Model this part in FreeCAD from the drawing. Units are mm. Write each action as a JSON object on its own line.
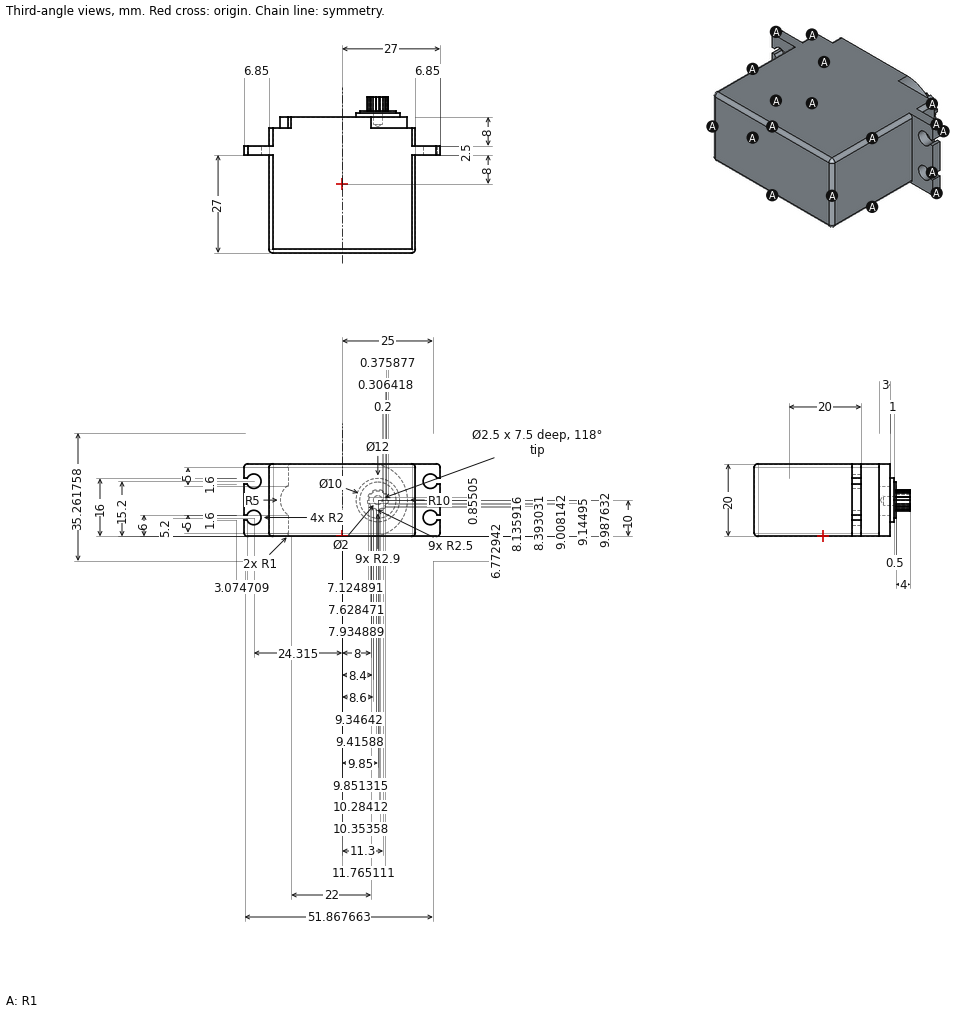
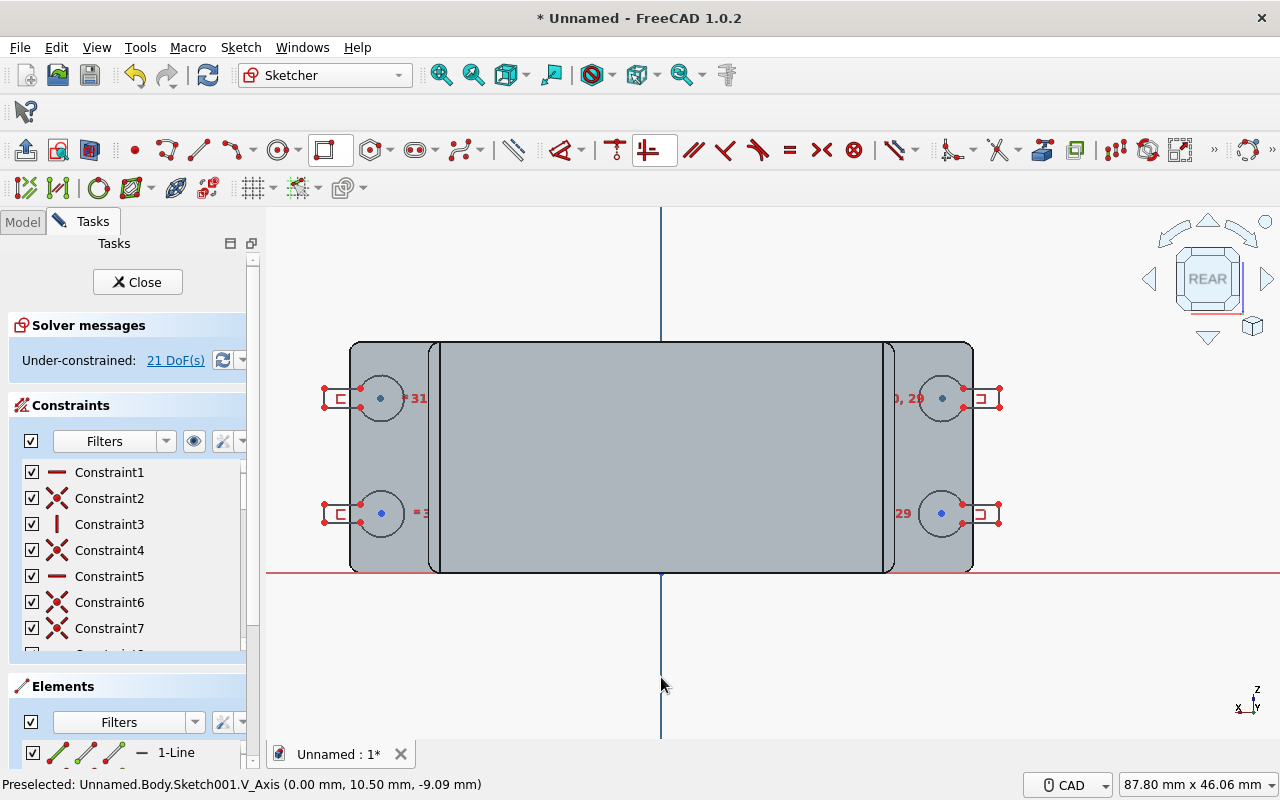
{"action": "left_click", "coordinate": [822, 150]}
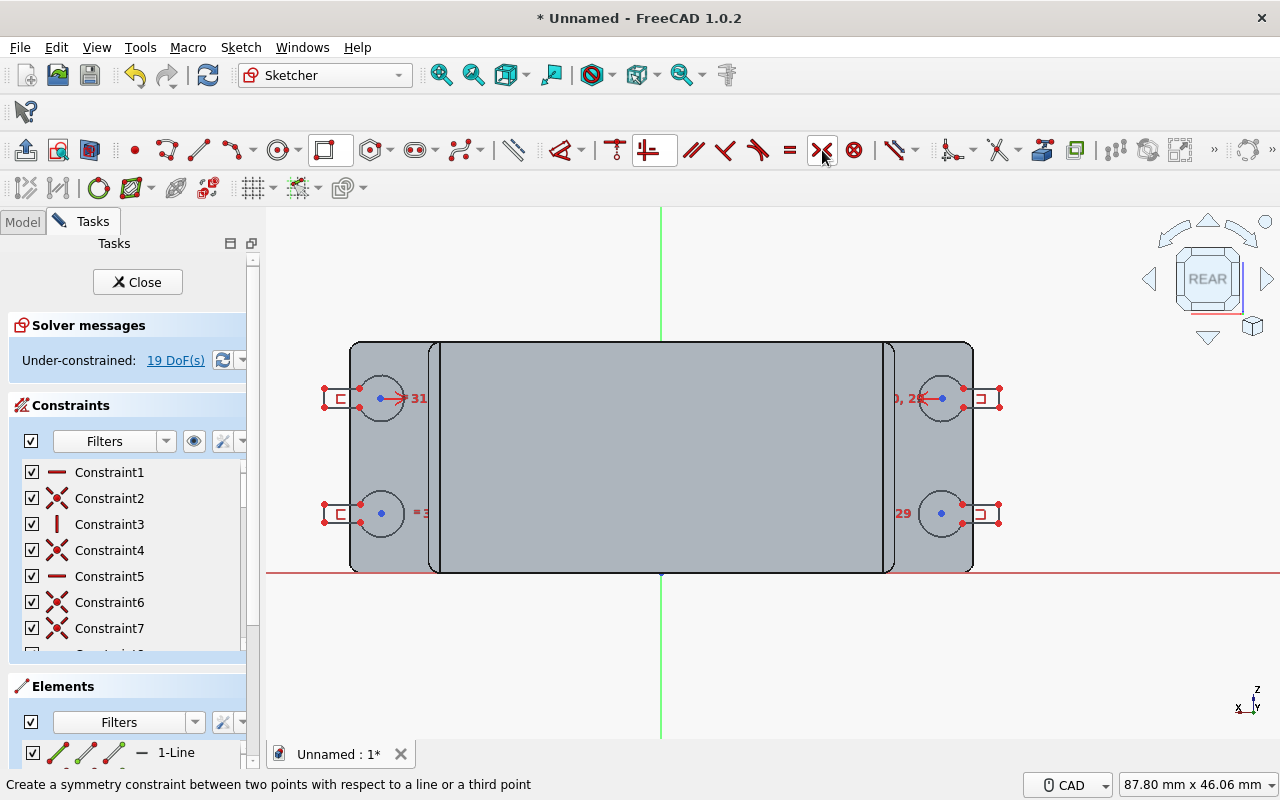
{"action": "left_click", "coordinate": [942, 514]}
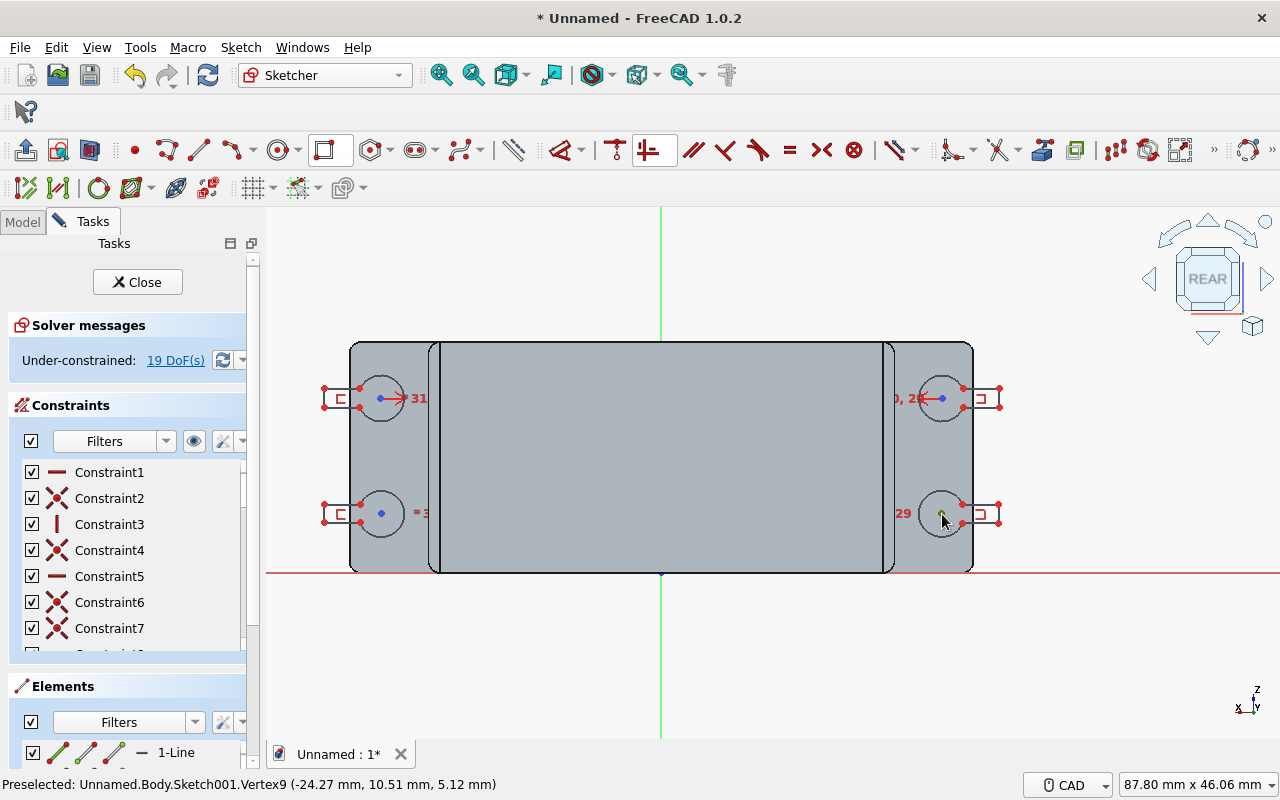
{"action": "left_click", "coordinate": [381, 514]}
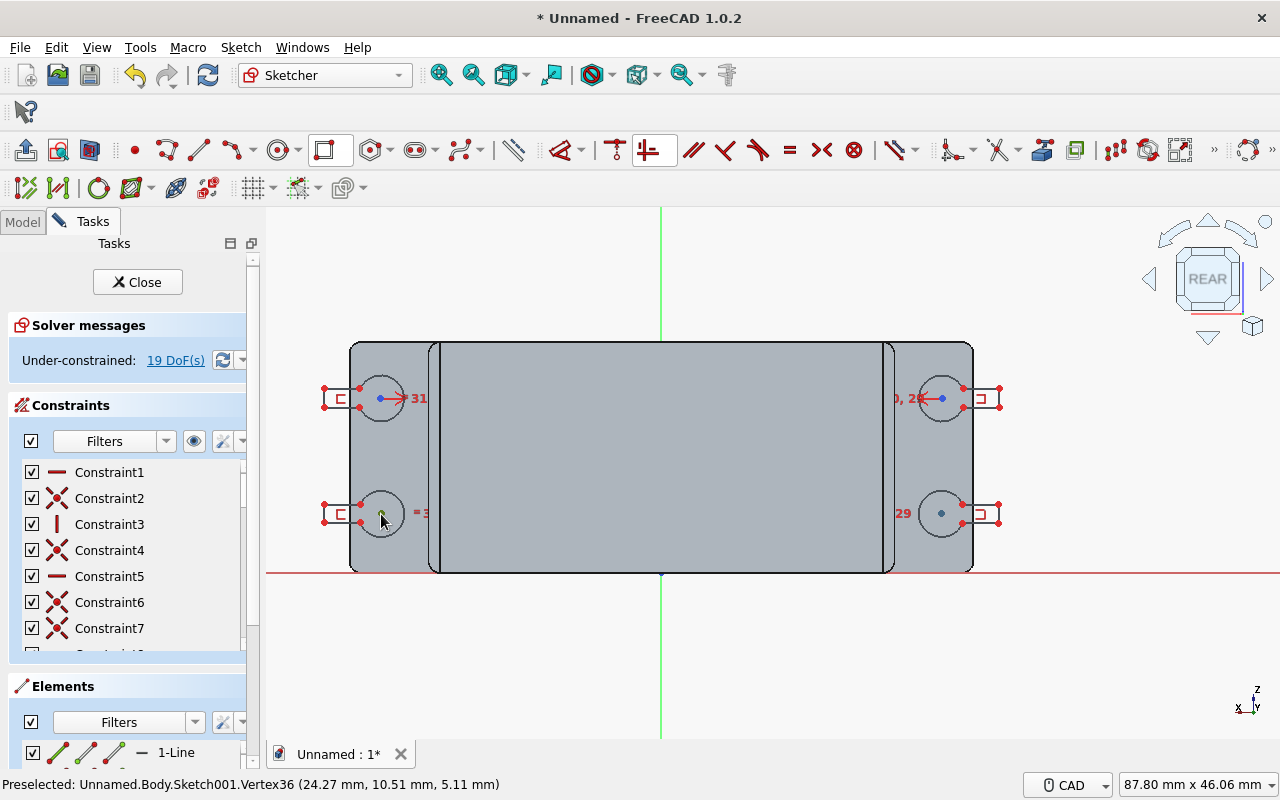
{"action": "left_click", "coordinate": [661, 677]}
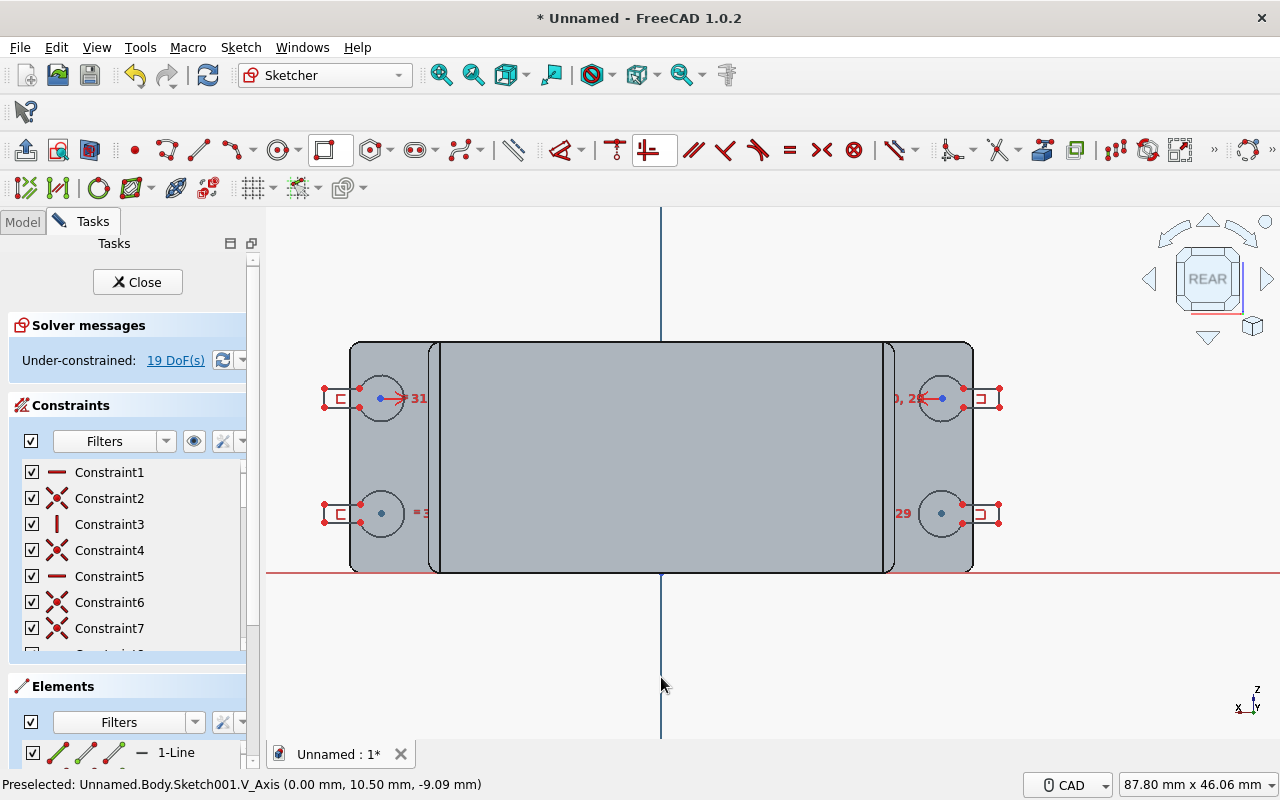
{"action": "left_click", "coordinate": [822, 150]}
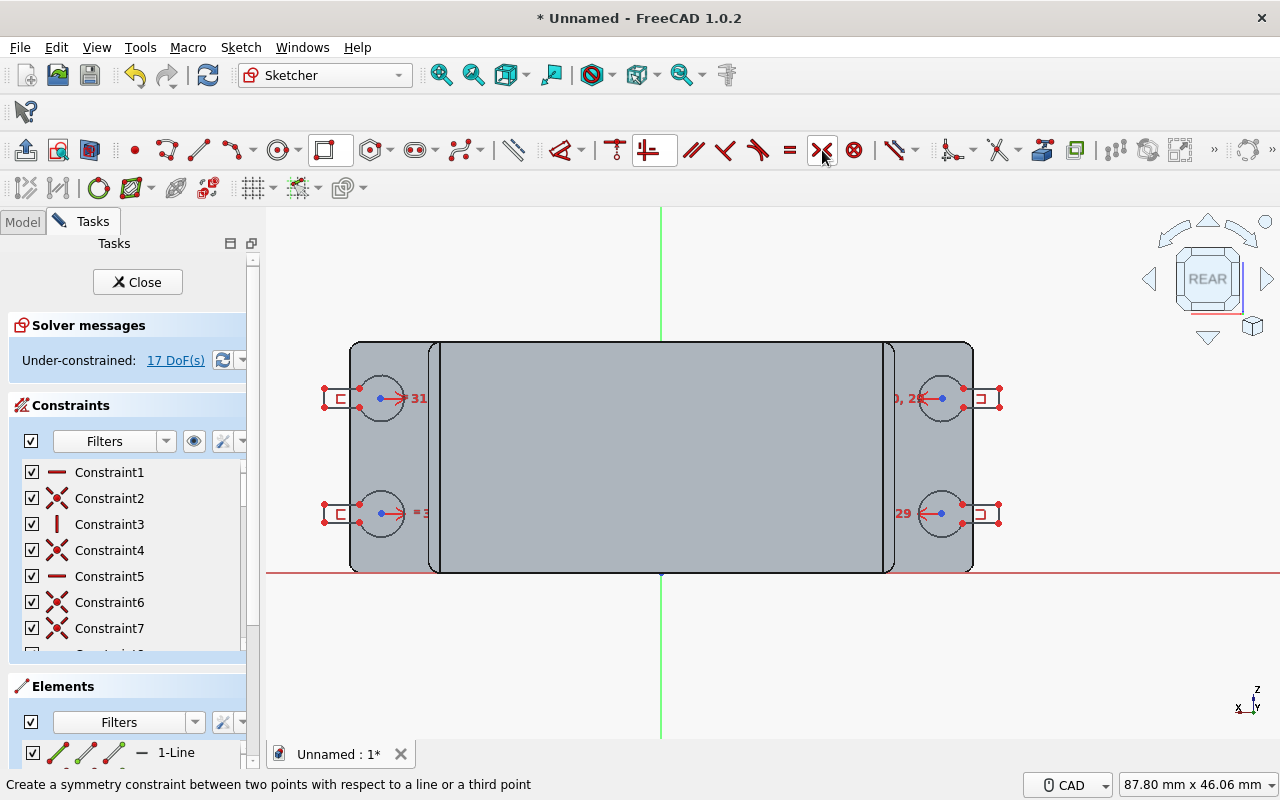
{"action": "left_click", "coordinate": [999, 389]}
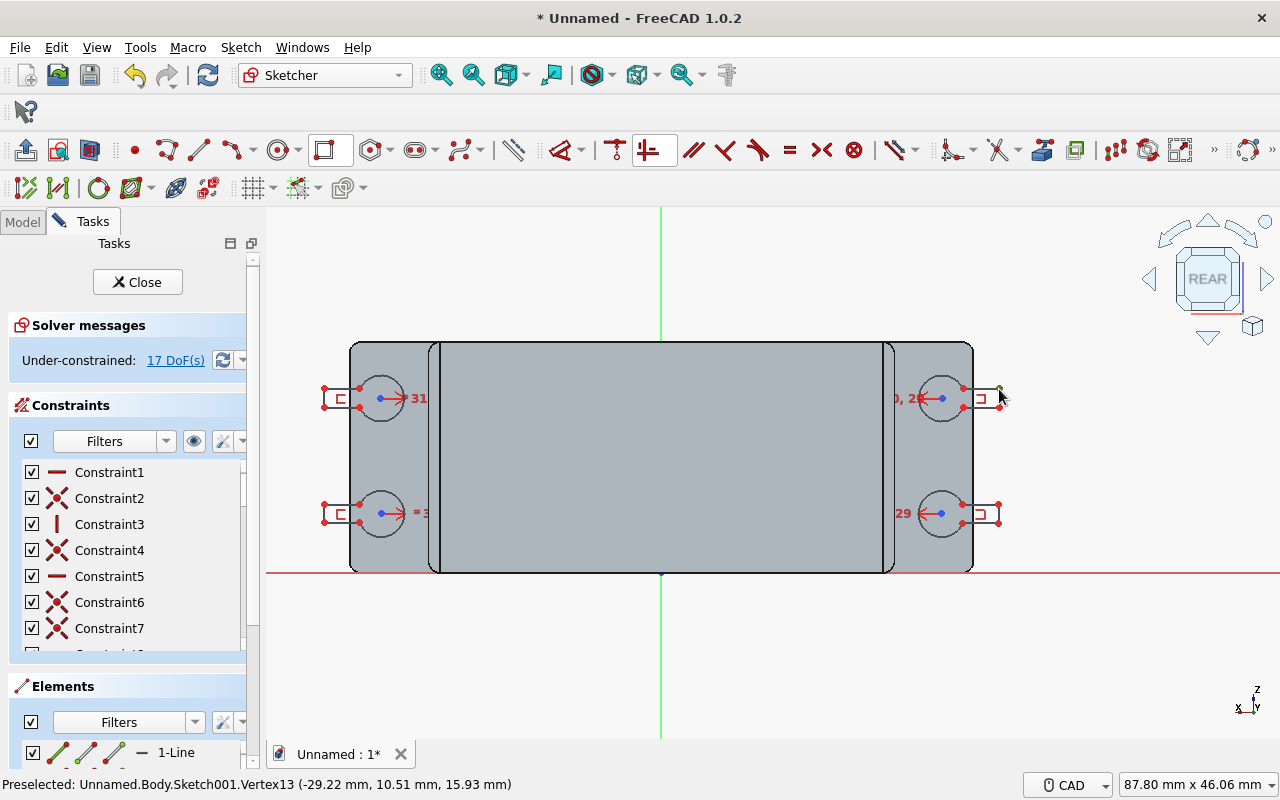
{"action": "left_click", "coordinate": [324, 389]}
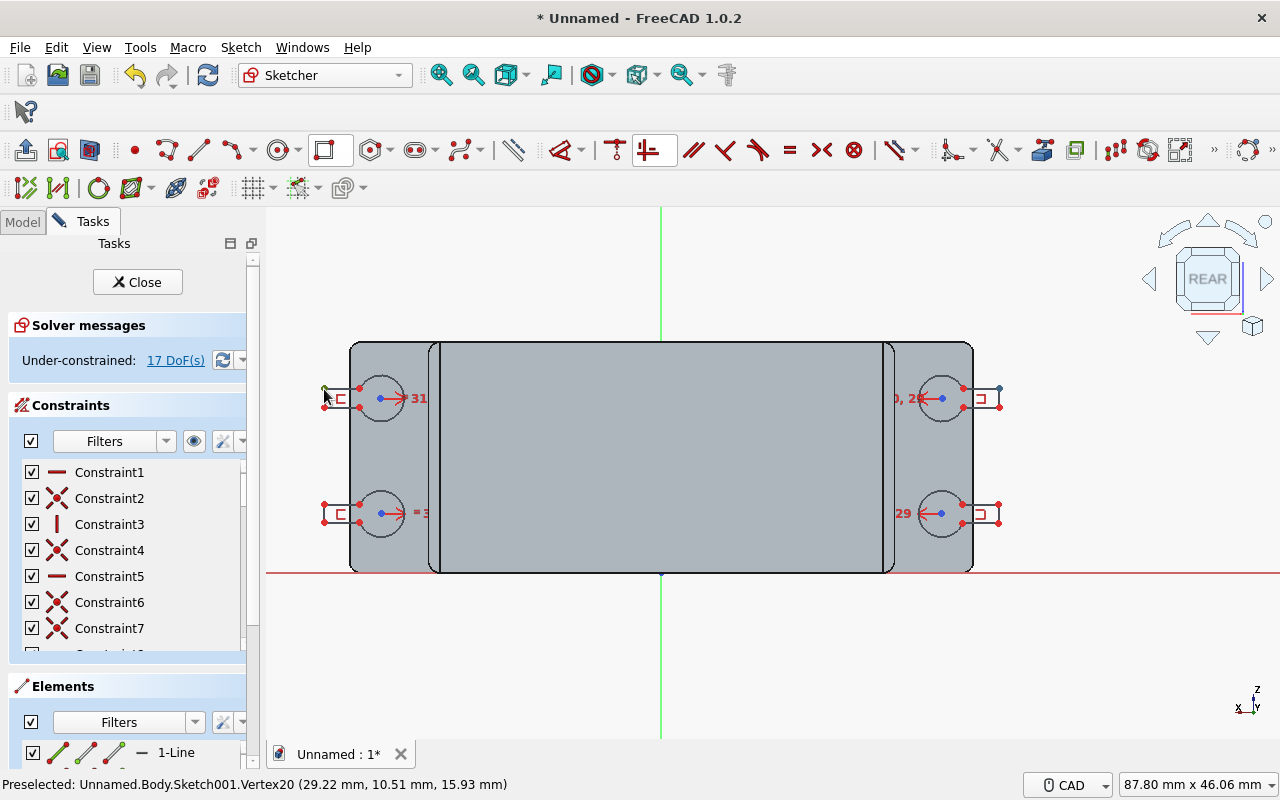
{"action": "left_click", "coordinate": [661, 677]}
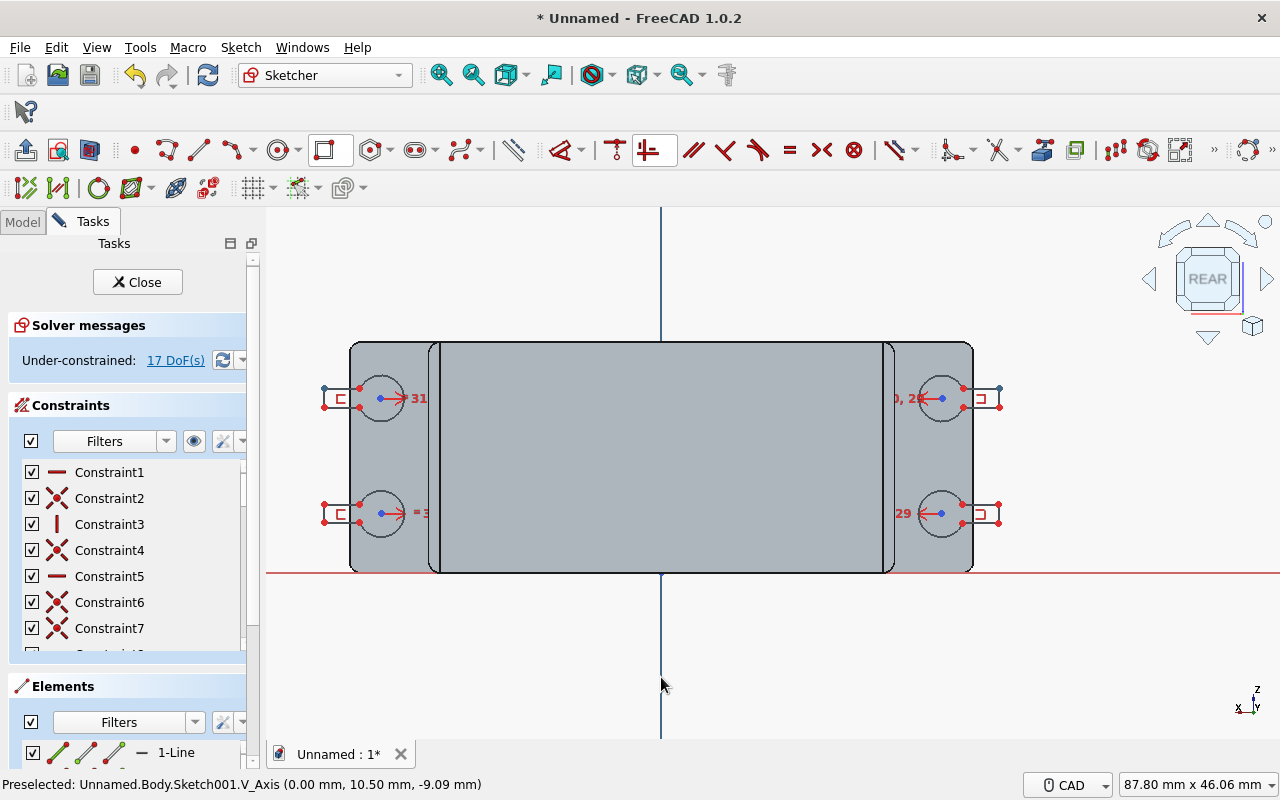
{"action": "key", "text": "s"}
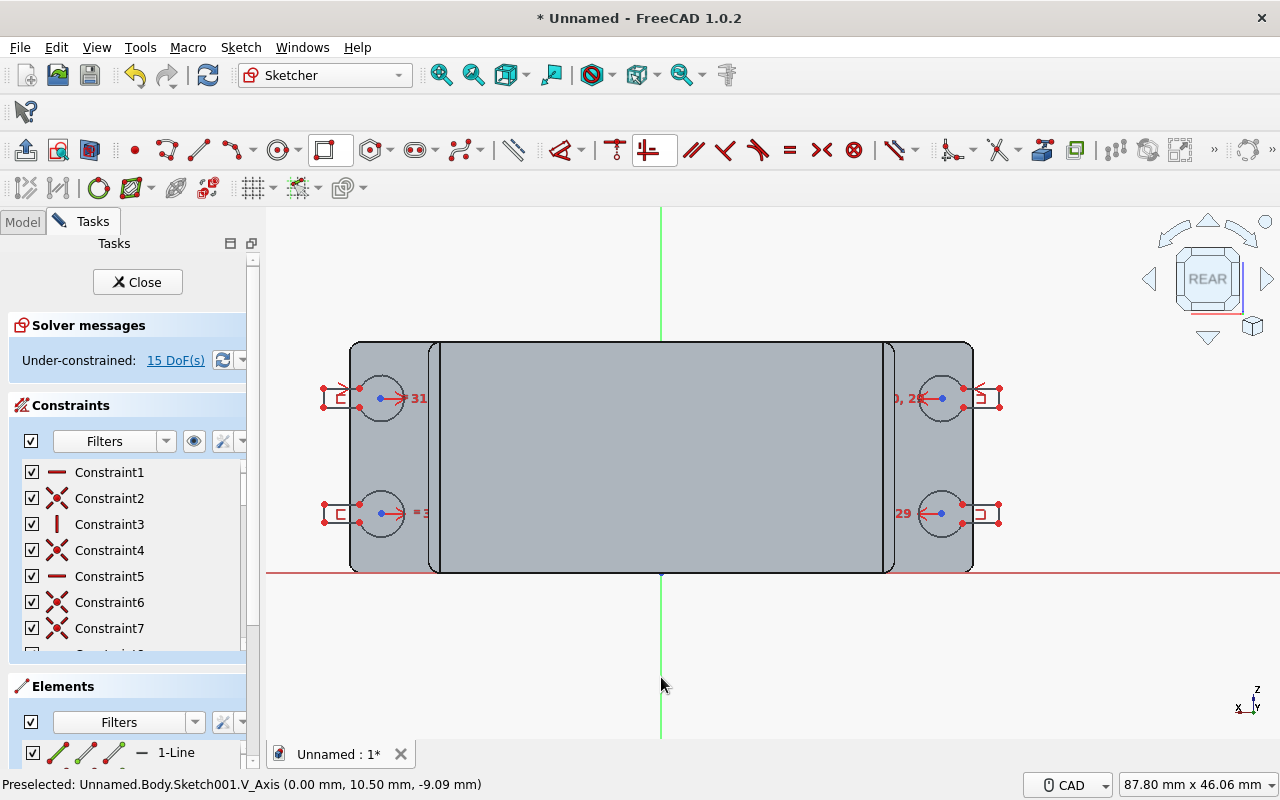
{"action": "left_click", "coordinate": [999, 505]}